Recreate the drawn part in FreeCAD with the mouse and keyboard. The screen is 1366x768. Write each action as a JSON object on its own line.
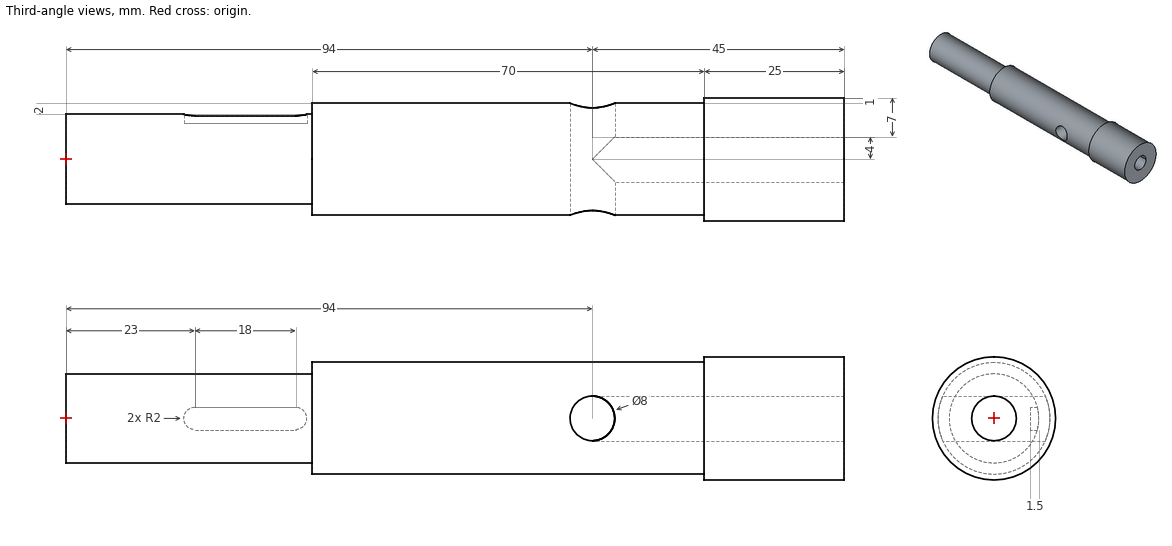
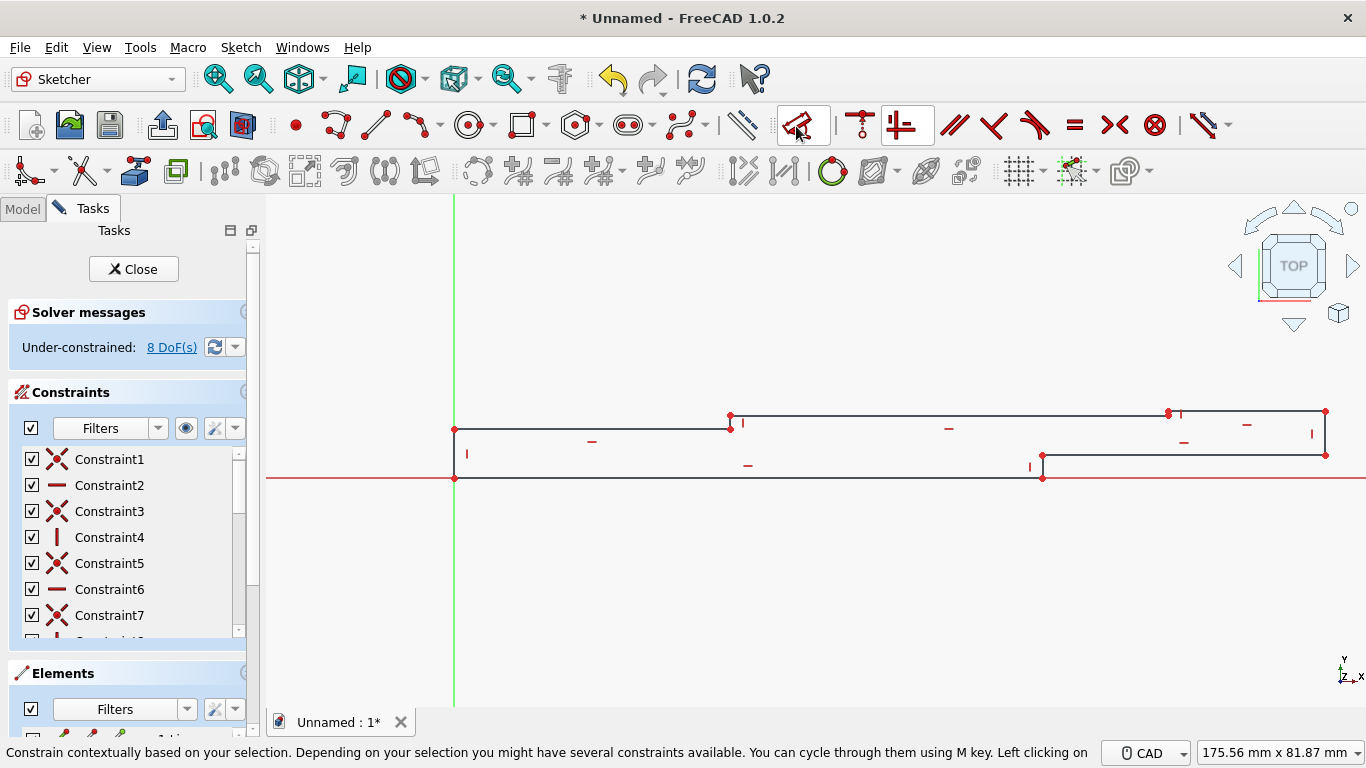
{"action": "scroll", "coordinate": [1043, 469], "scroll_direction": "up", "scroll_amount": 3}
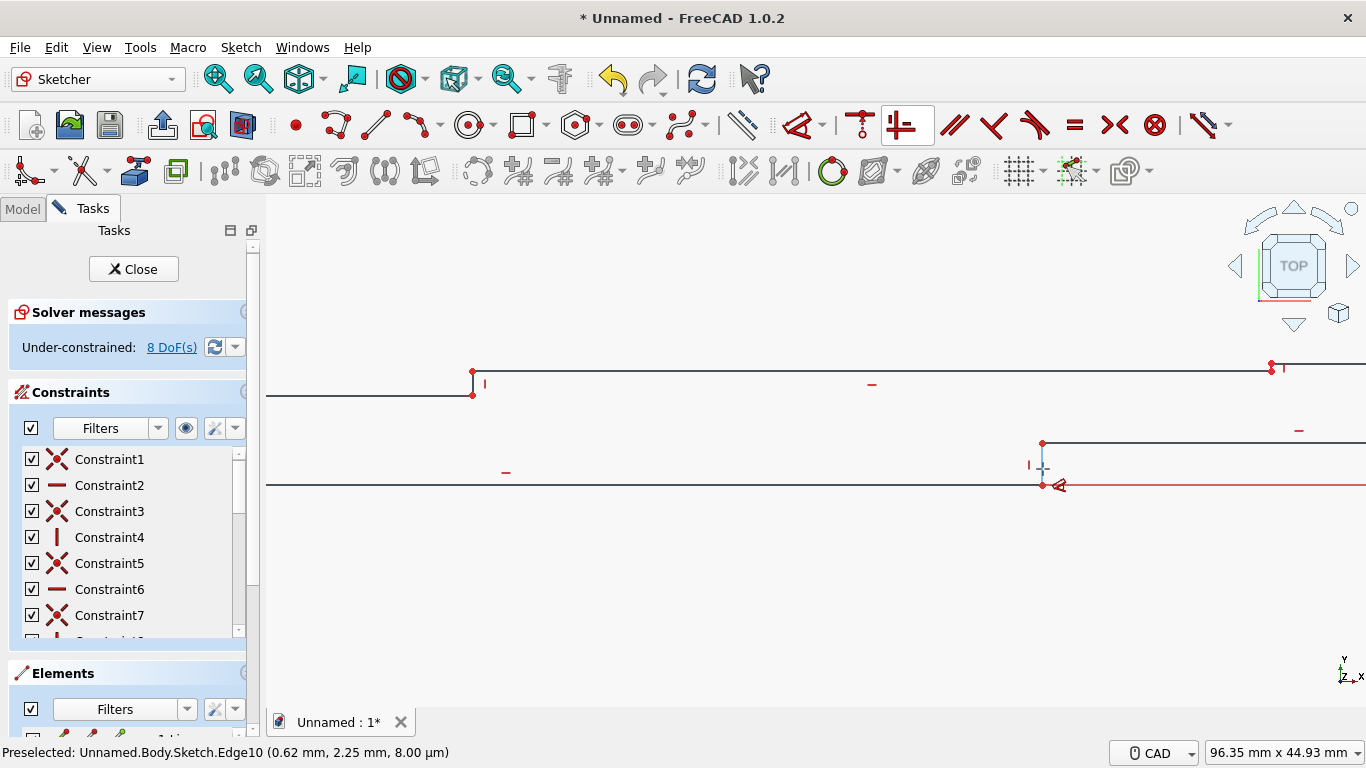
{"action": "left_click", "coordinate": [1042, 468]}
{"action": "left_click", "coordinate": [1076, 464]}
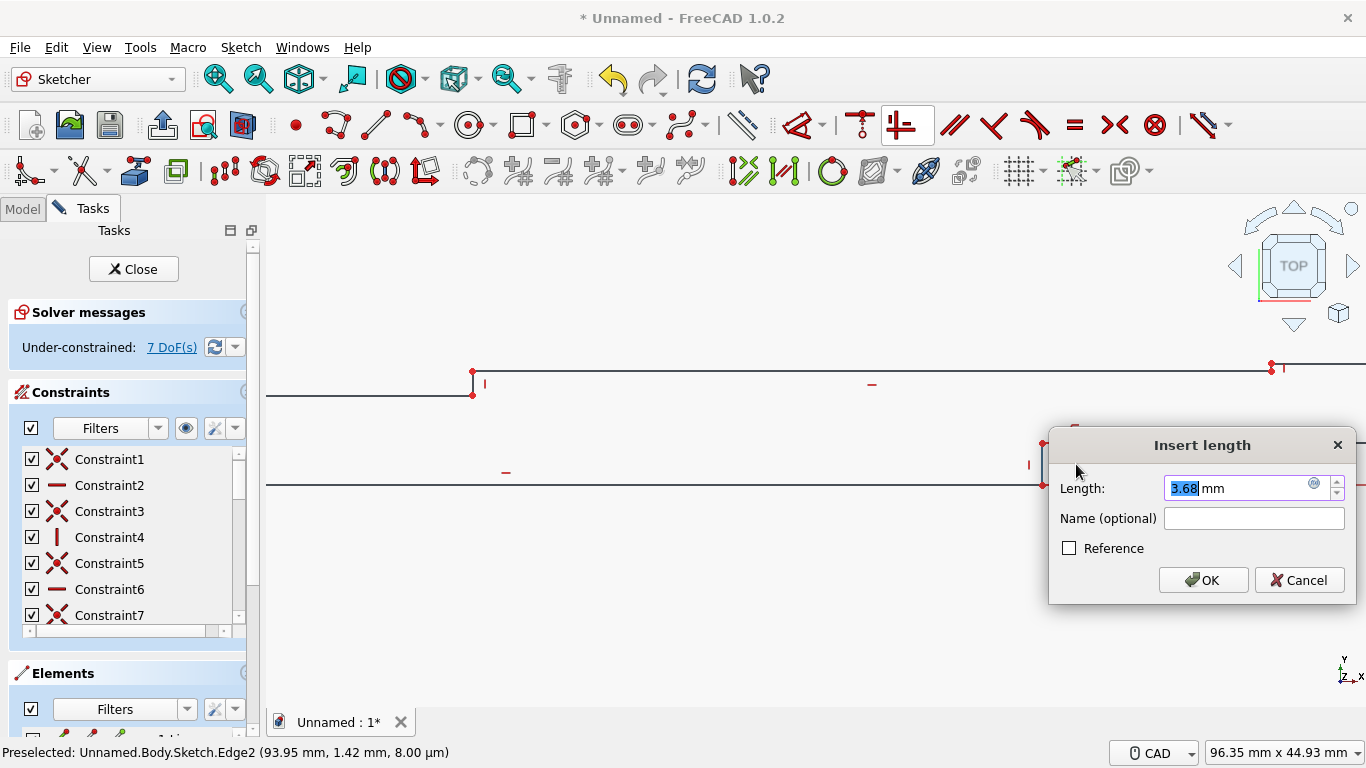
{"action": "type", "text": "4"}
{"action": "key", "text": "Return"}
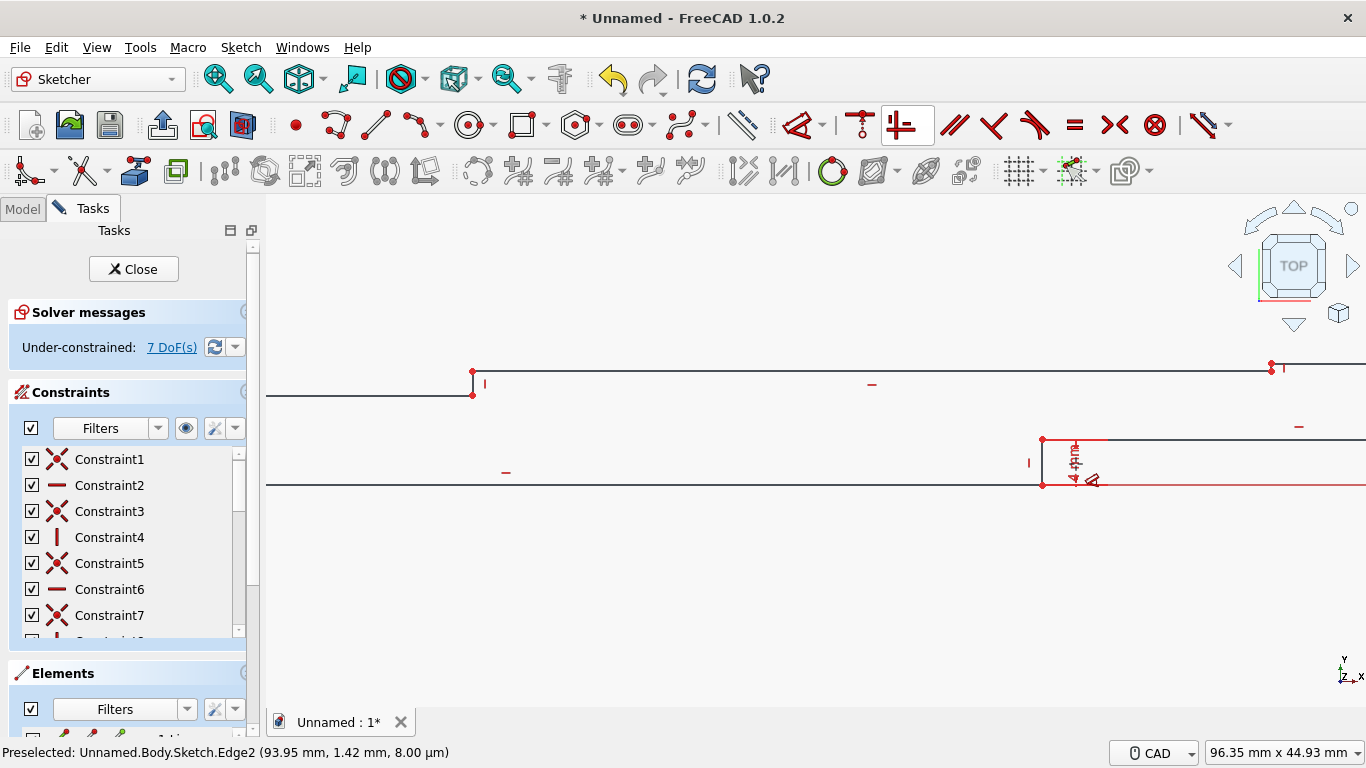
{"action": "scroll", "coordinate": [738, 467], "scroll_direction": "down", "scroll_amount": 5}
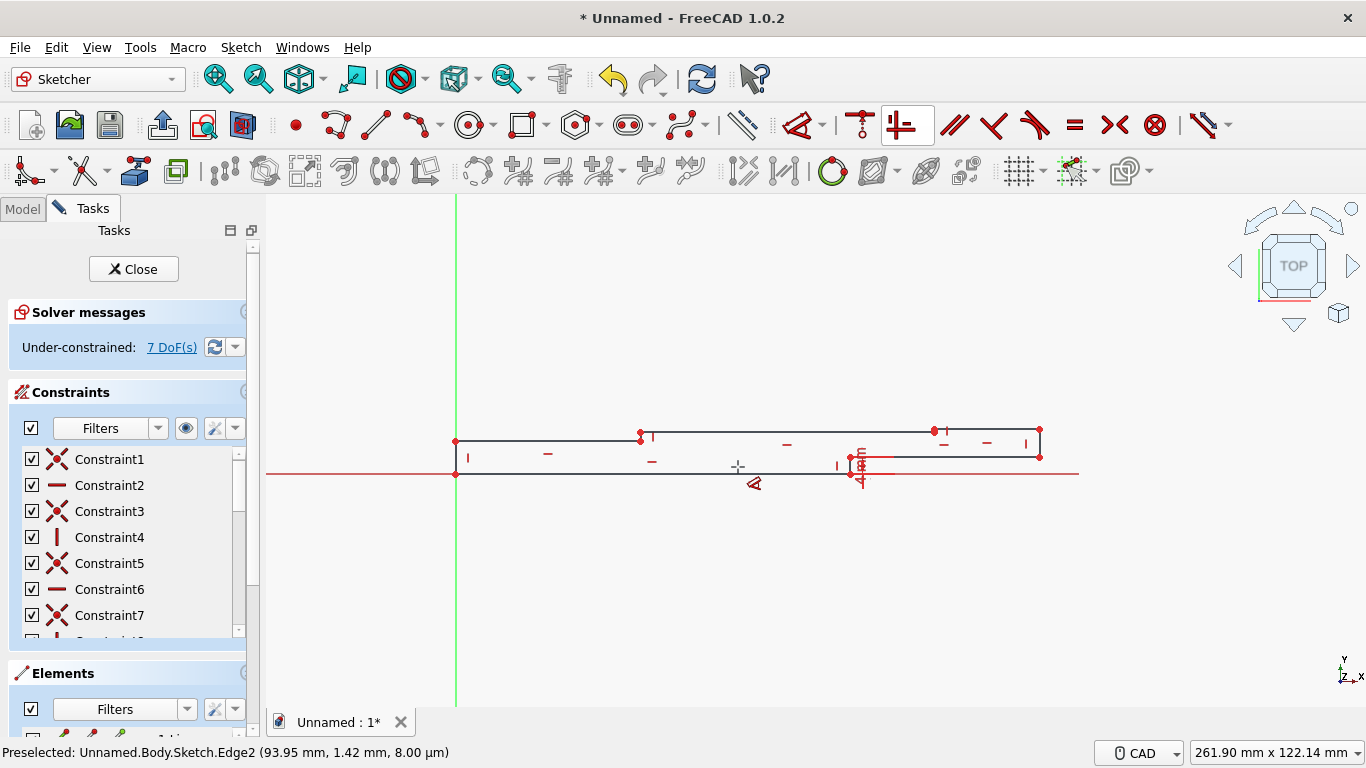
{"action": "scroll", "coordinate": [1040, 449], "scroll_direction": "up", "scroll_amount": 3}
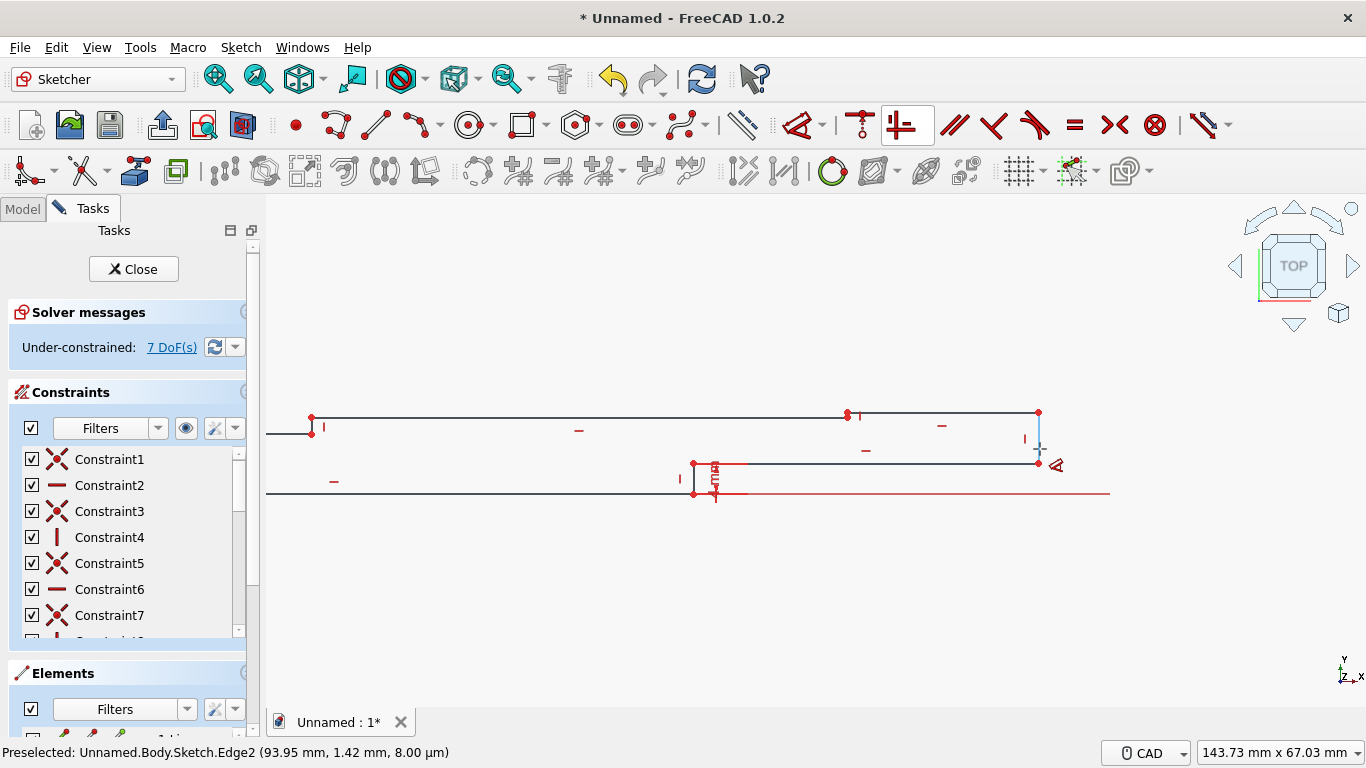
{"action": "left_click", "coordinate": [1039, 448]}
{"action": "left_click", "coordinate": [1073, 438]}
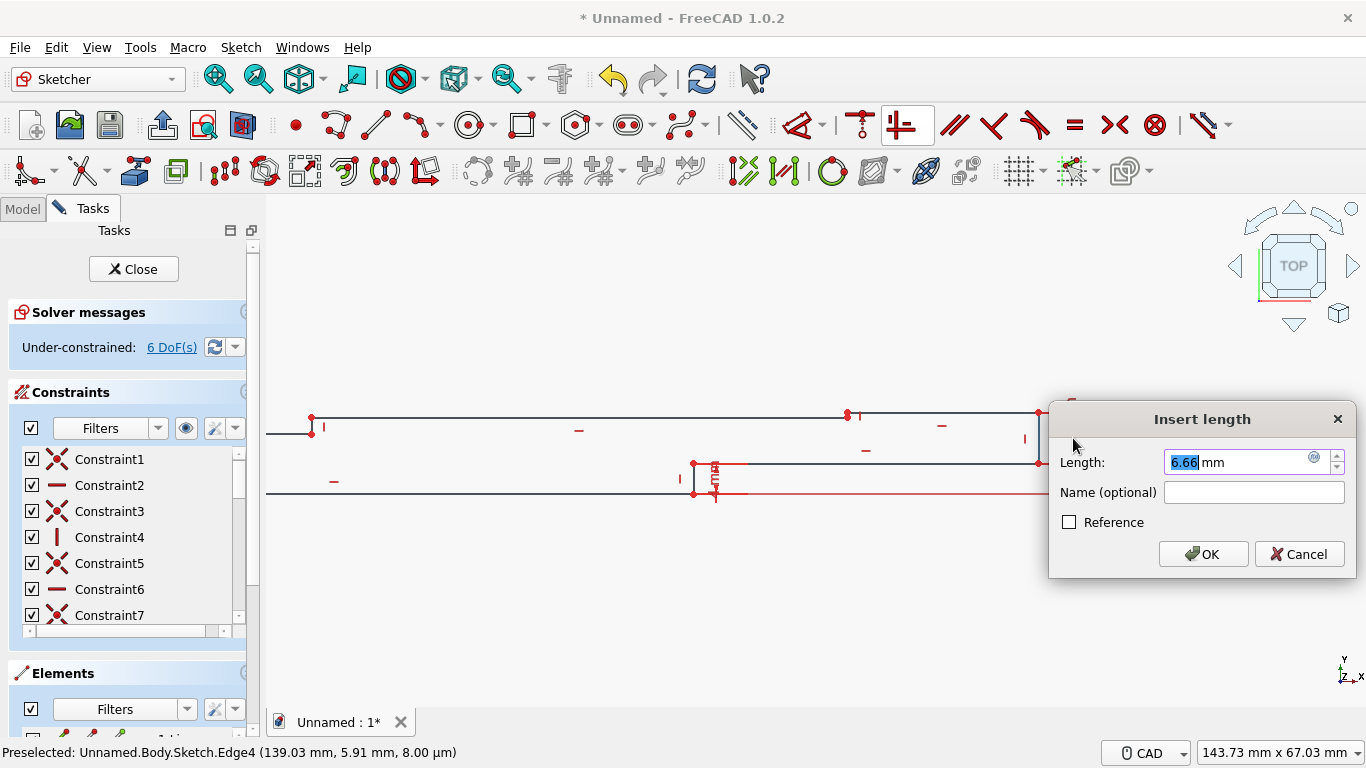
{"action": "type", "text": "7"}
{"action": "key", "text": "Return"}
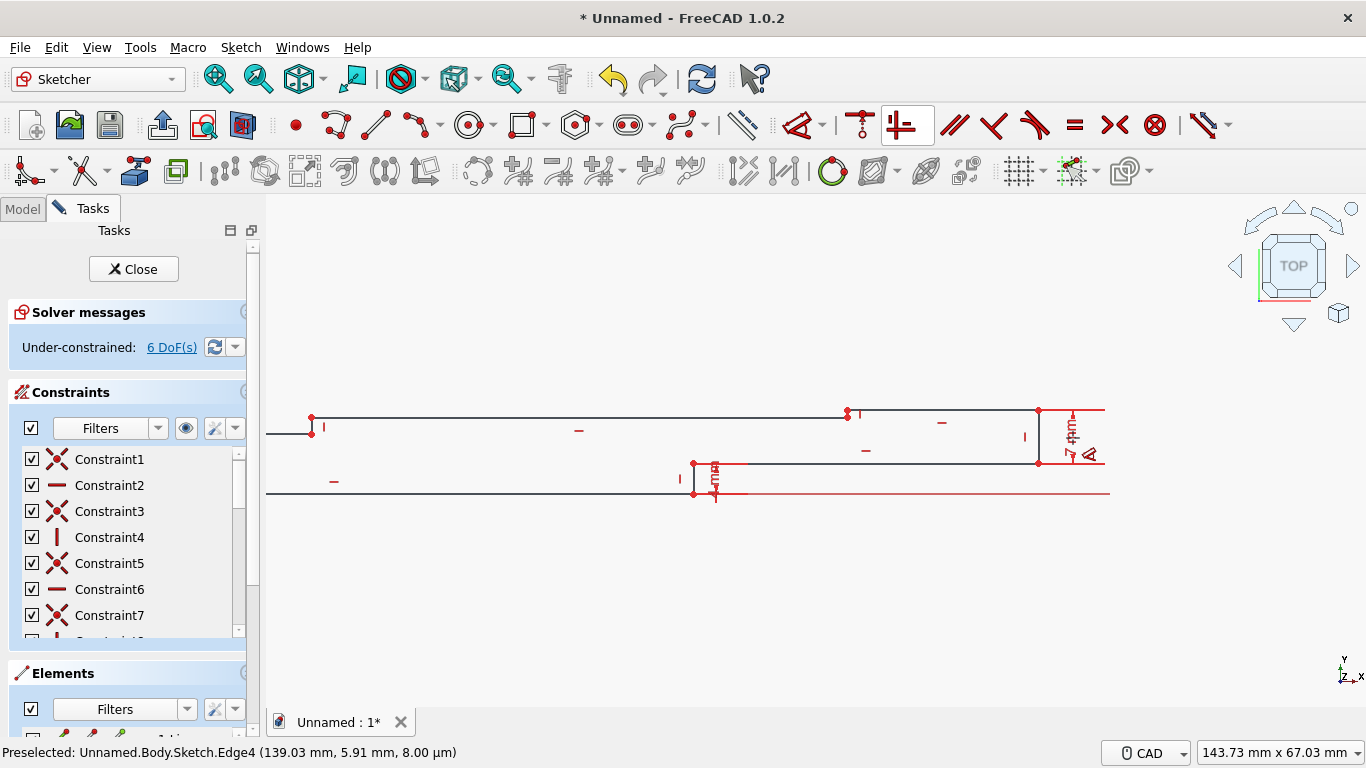
{"action": "scroll", "coordinate": [847, 414], "scroll_direction": "up", "scroll_amount": 9}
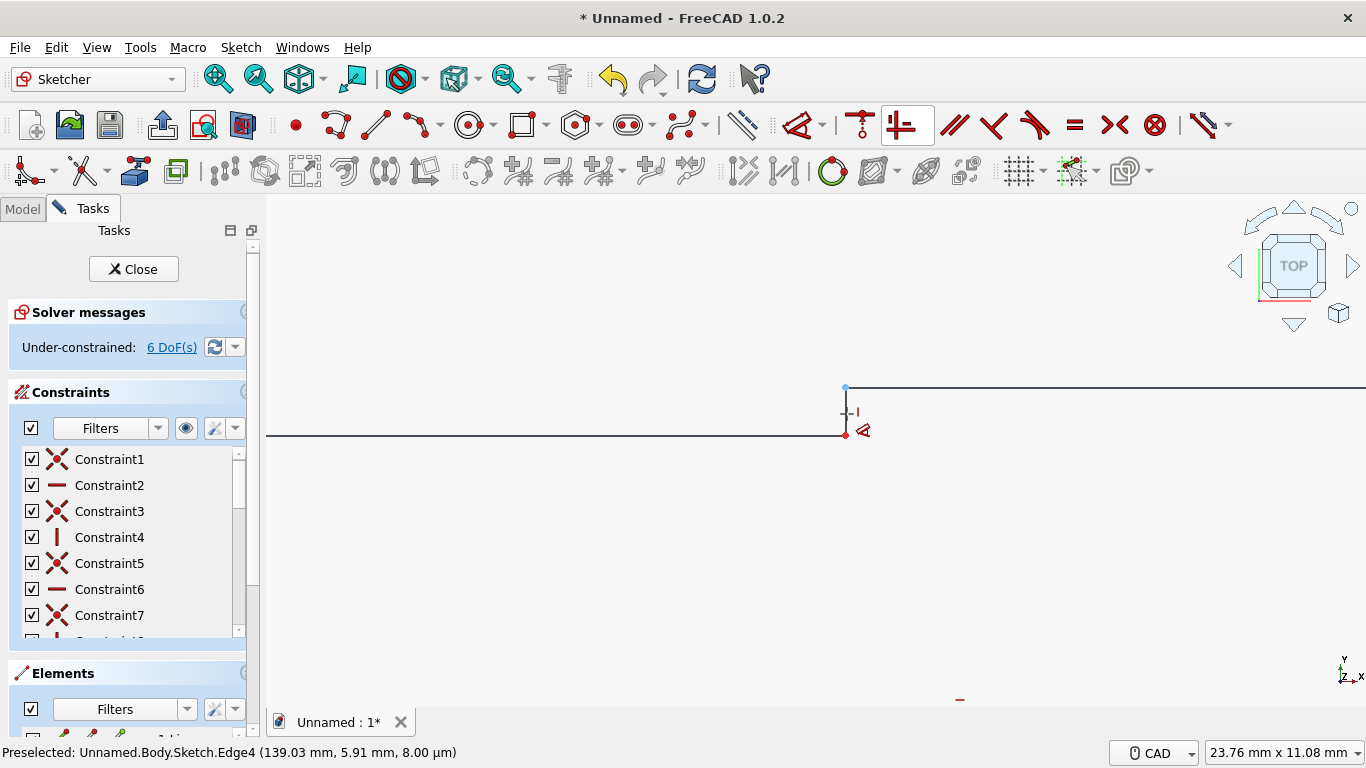
{"action": "left_click", "coordinate": [846, 412]}
{"action": "left_click", "coordinate": [880, 412]}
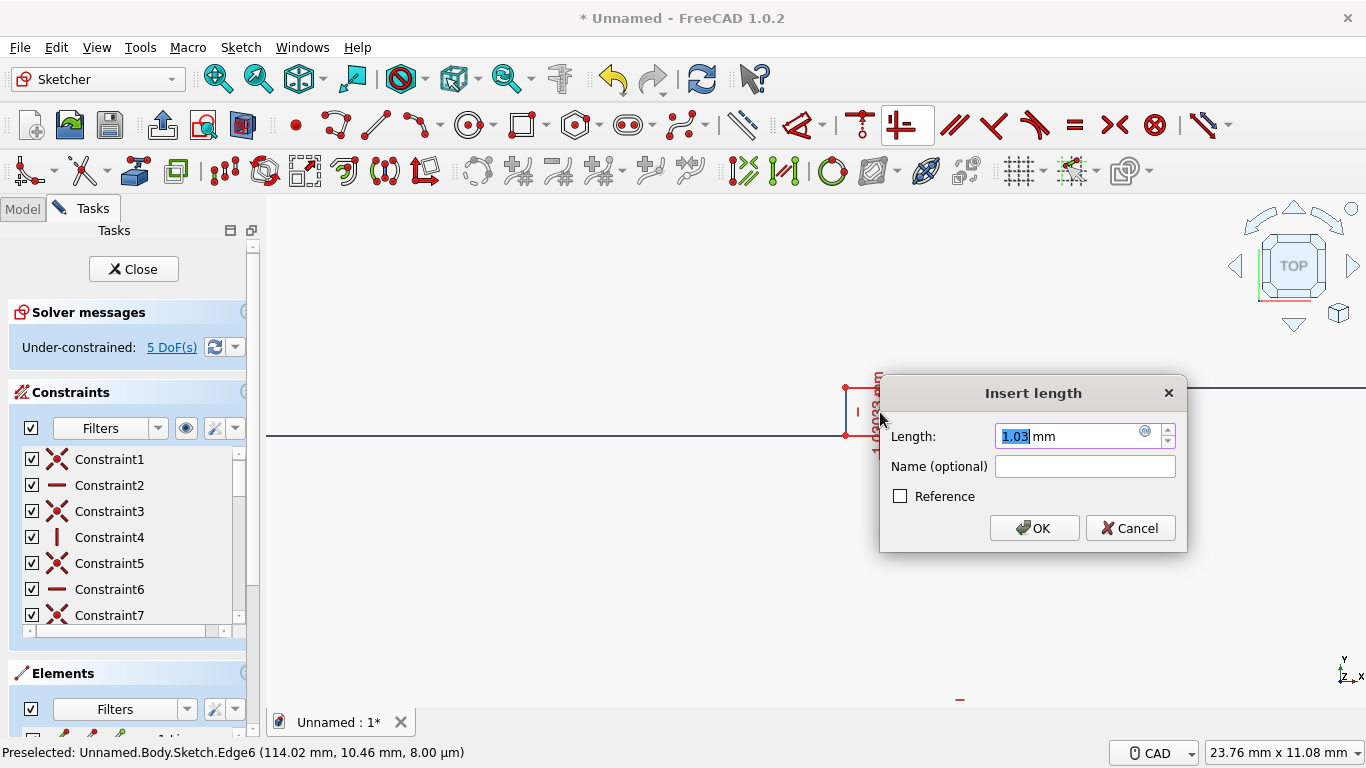
{"action": "type", "text": "1"}
{"action": "key", "text": "Return"}